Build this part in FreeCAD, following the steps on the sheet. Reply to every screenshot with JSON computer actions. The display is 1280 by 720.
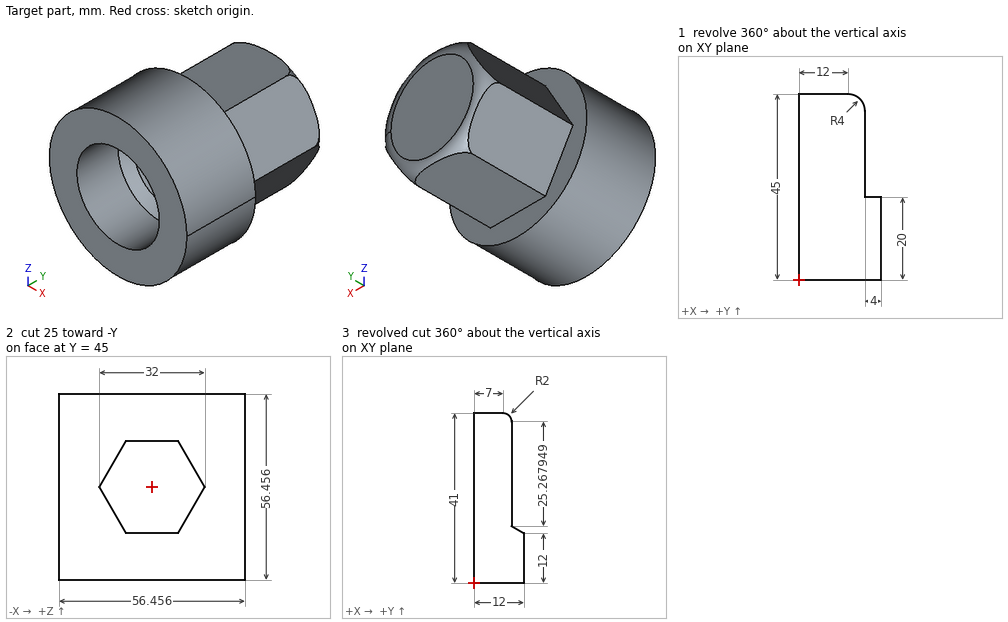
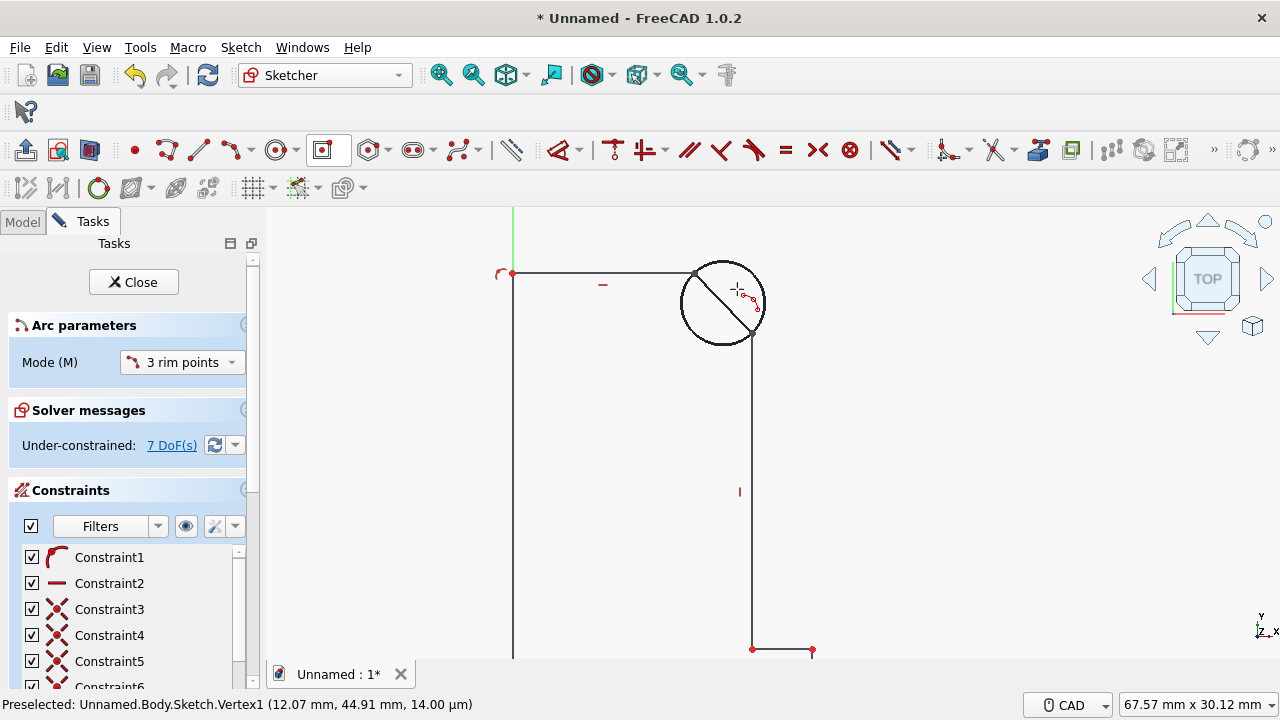
{"action": "left_click", "coordinate": [736, 289]}
{"action": "key", "text": "Escape"}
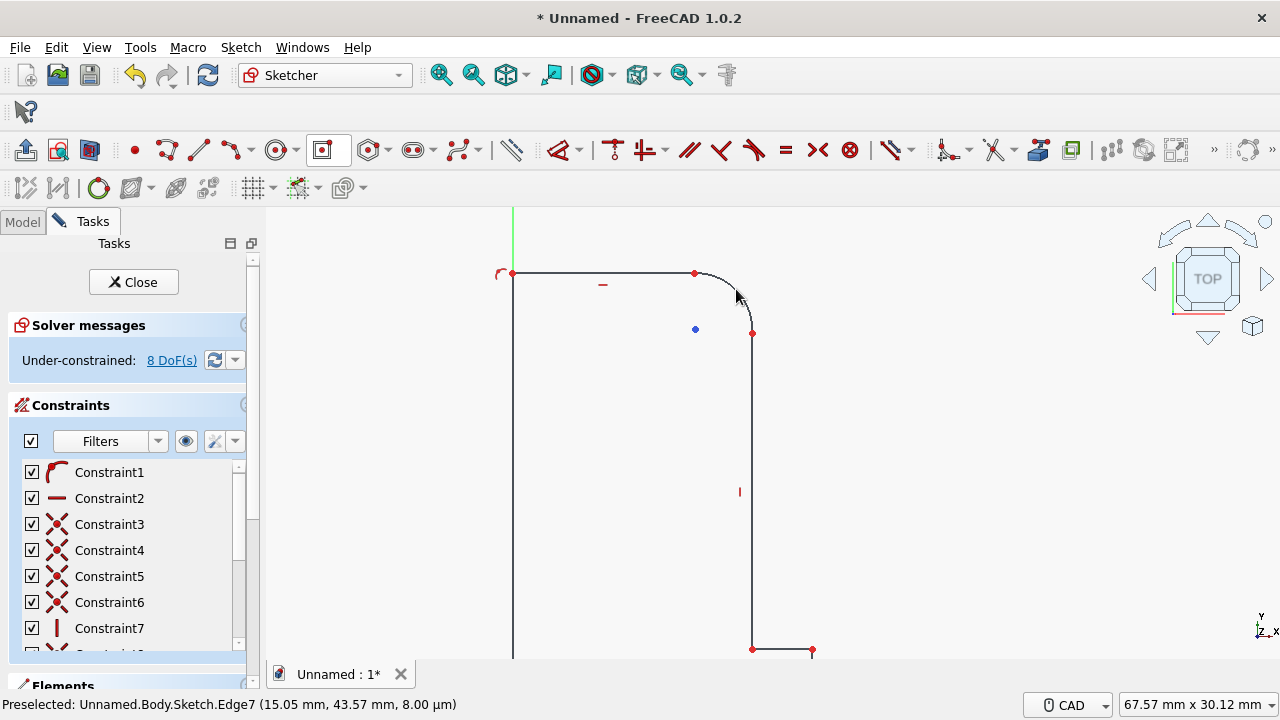
{"action": "left_click", "coordinate": [640, 273]}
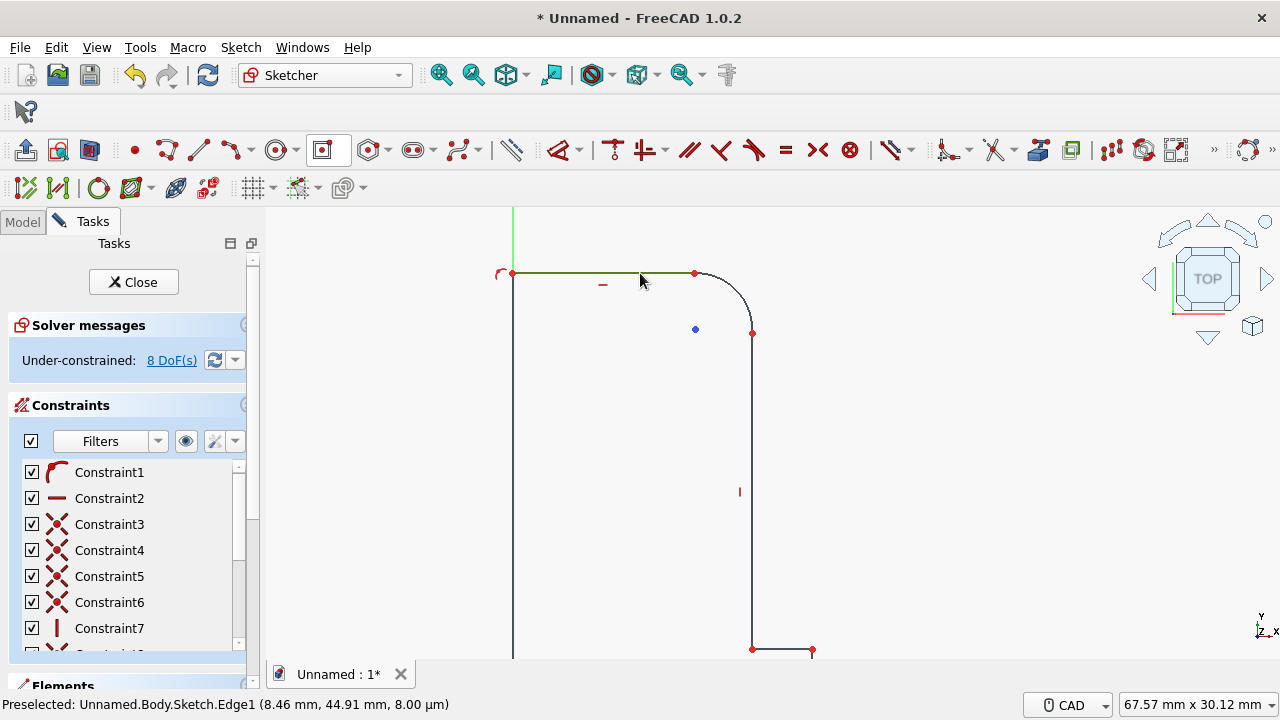
{"action": "left_click", "coordinate": [747, 306]}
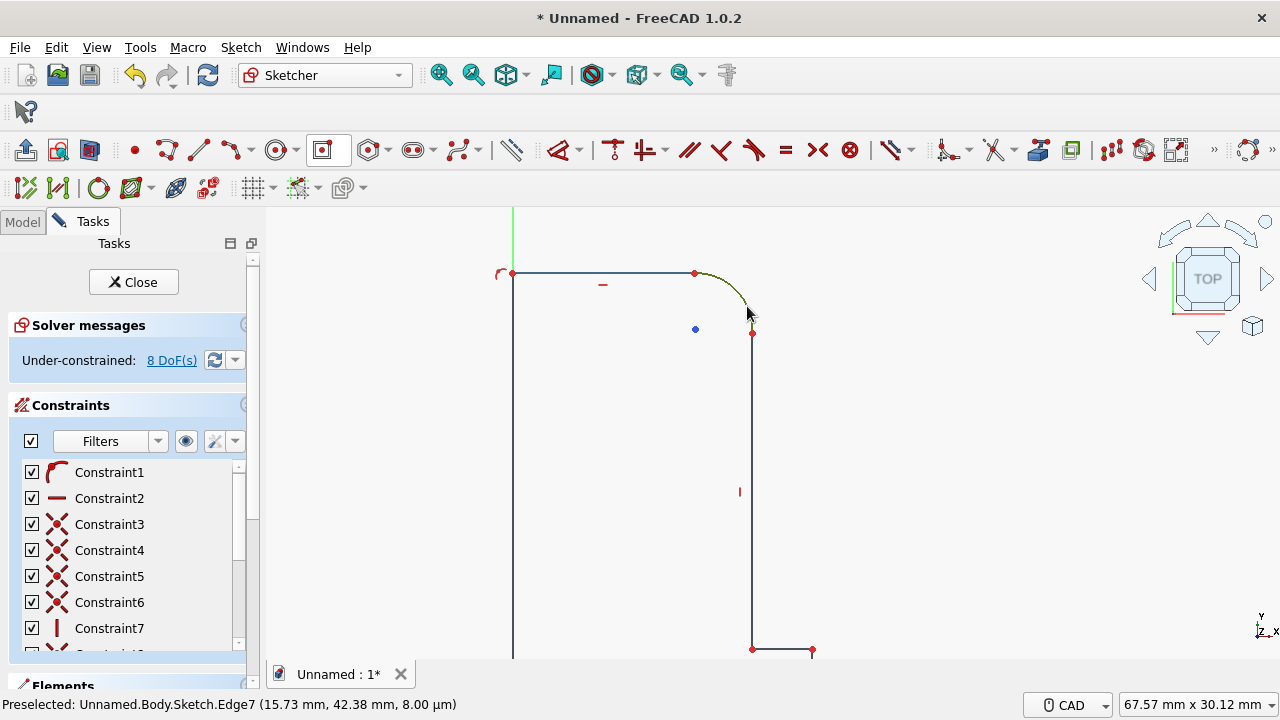
{"action": "key", "text": "t"}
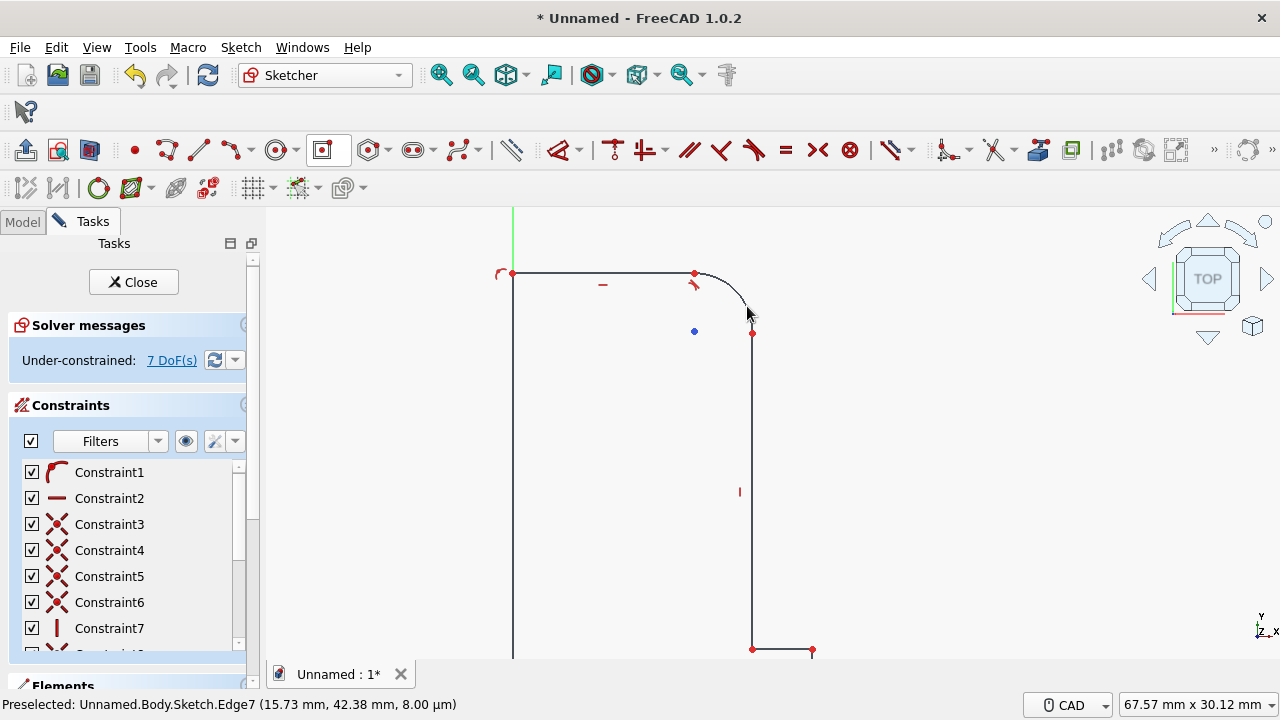
{"action": "left_click", "coordinate": [752, 555]}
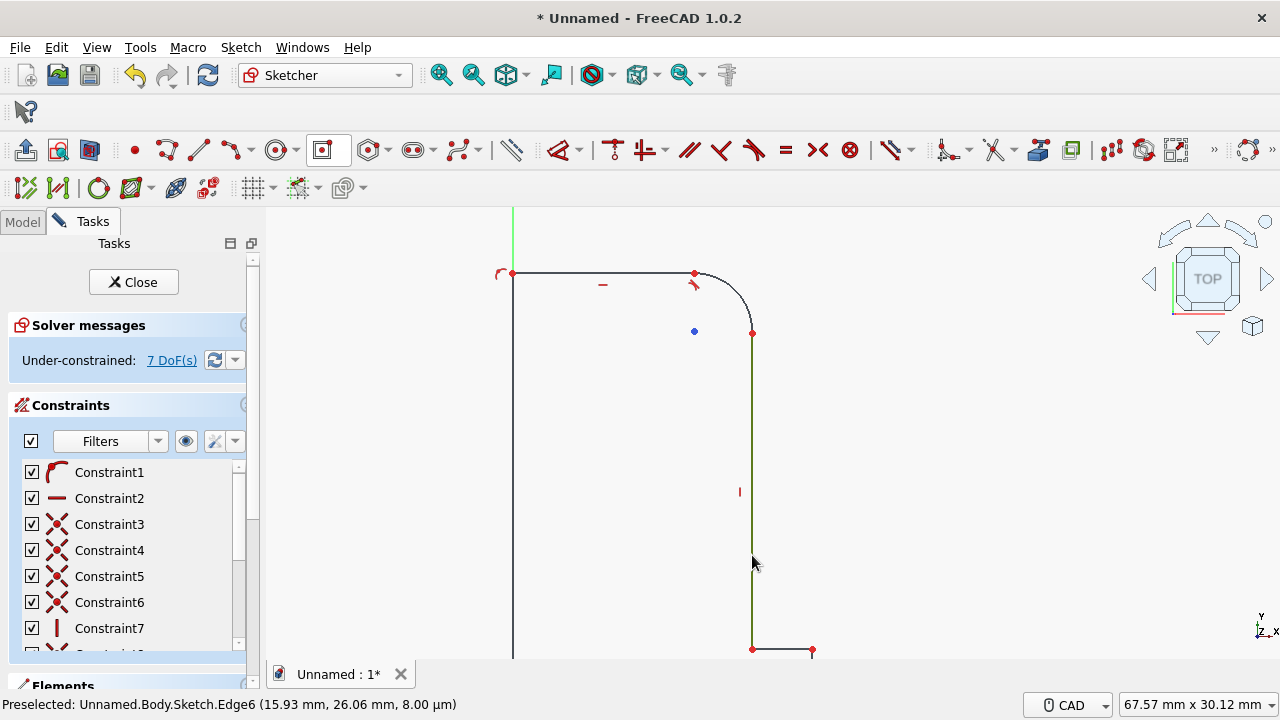
{"action": "left_click", "coordinate": [746, 306]}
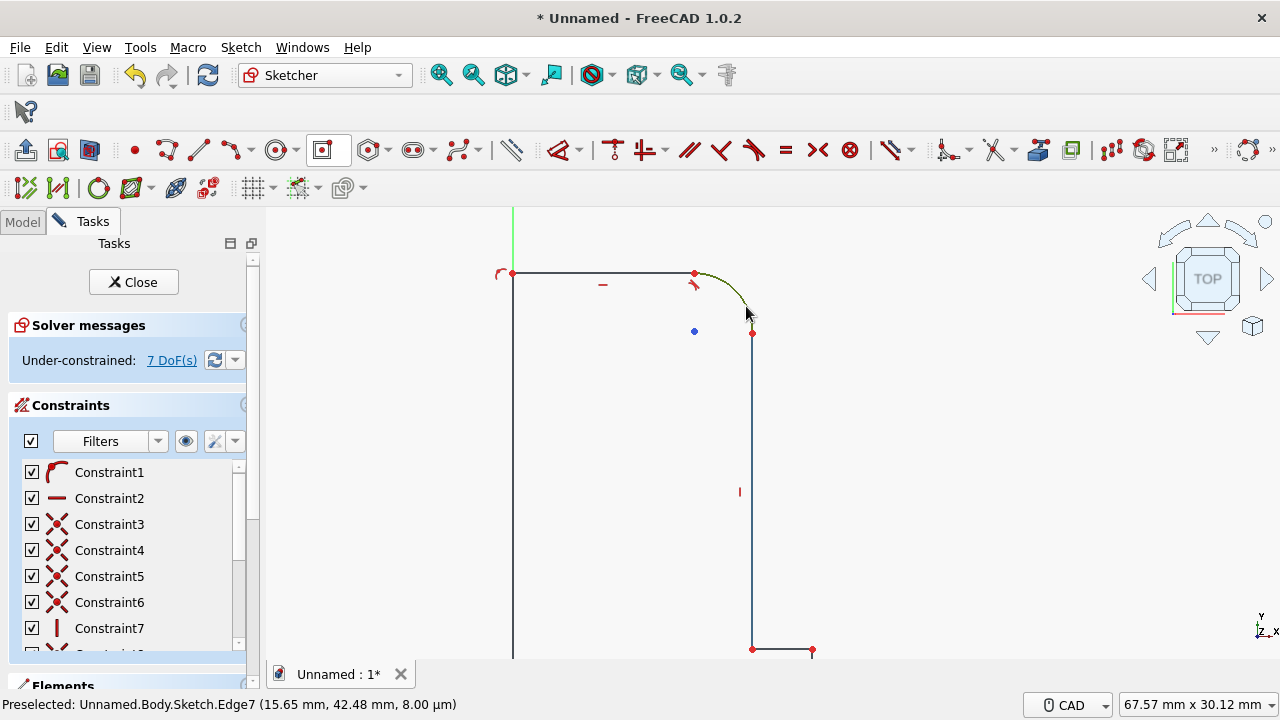
{"action": "key", "text": "t"}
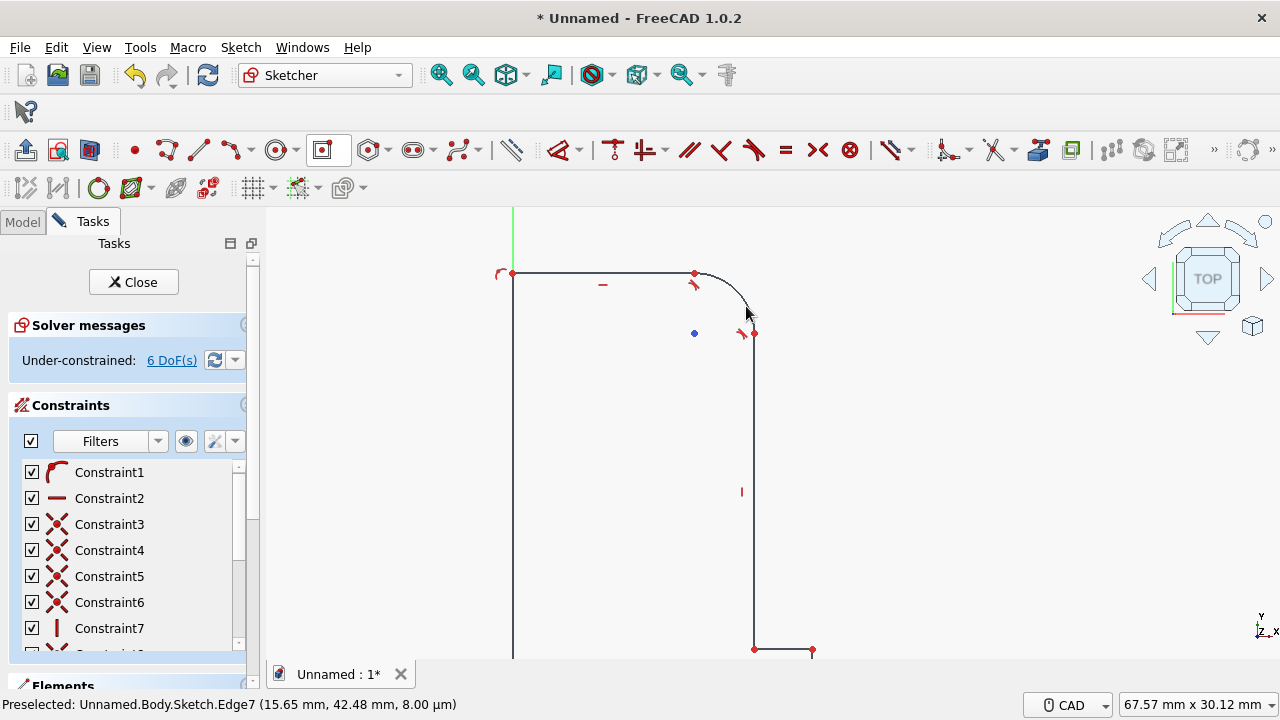
{"action": "scroll", "coordinate": [738, 289], "scroll_direction": "down", "scroll_amount": 4}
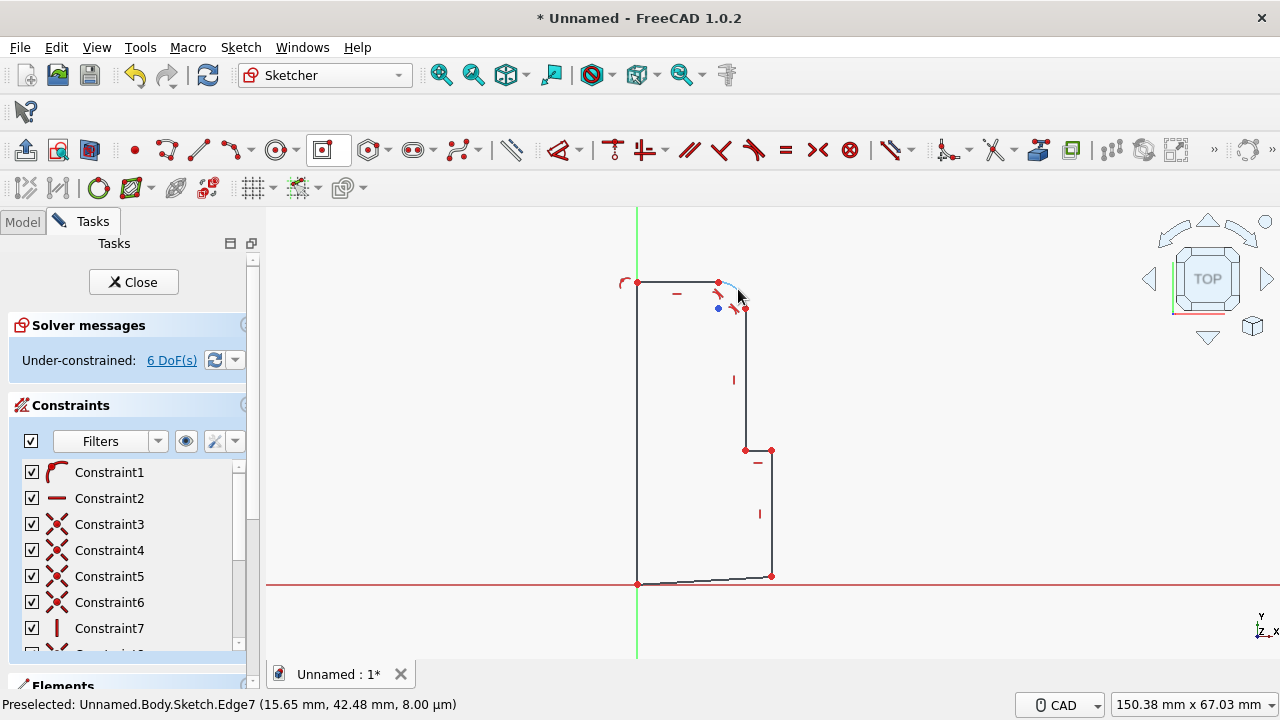
{"action": "scroll", "coordinate": [731, 579], "scroll_direction": "up", "scroll_amount": 5}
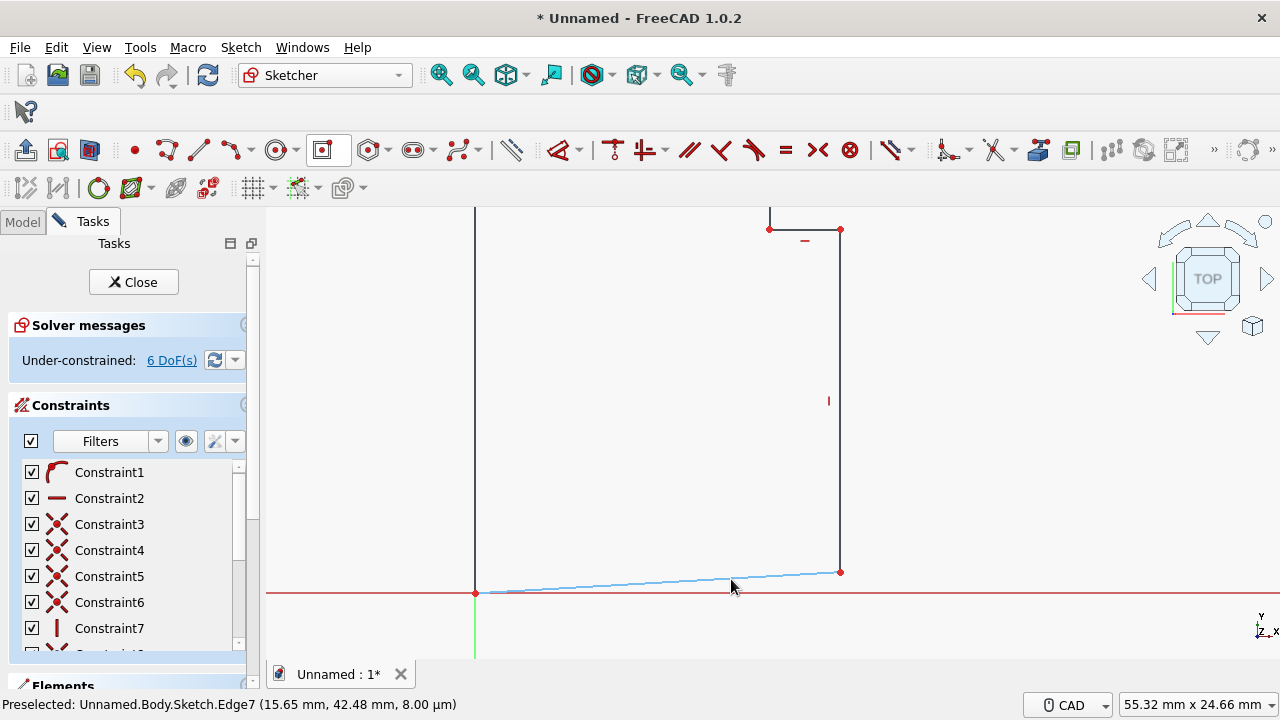
{"action": "left_click", "coordinate": [731, 579]}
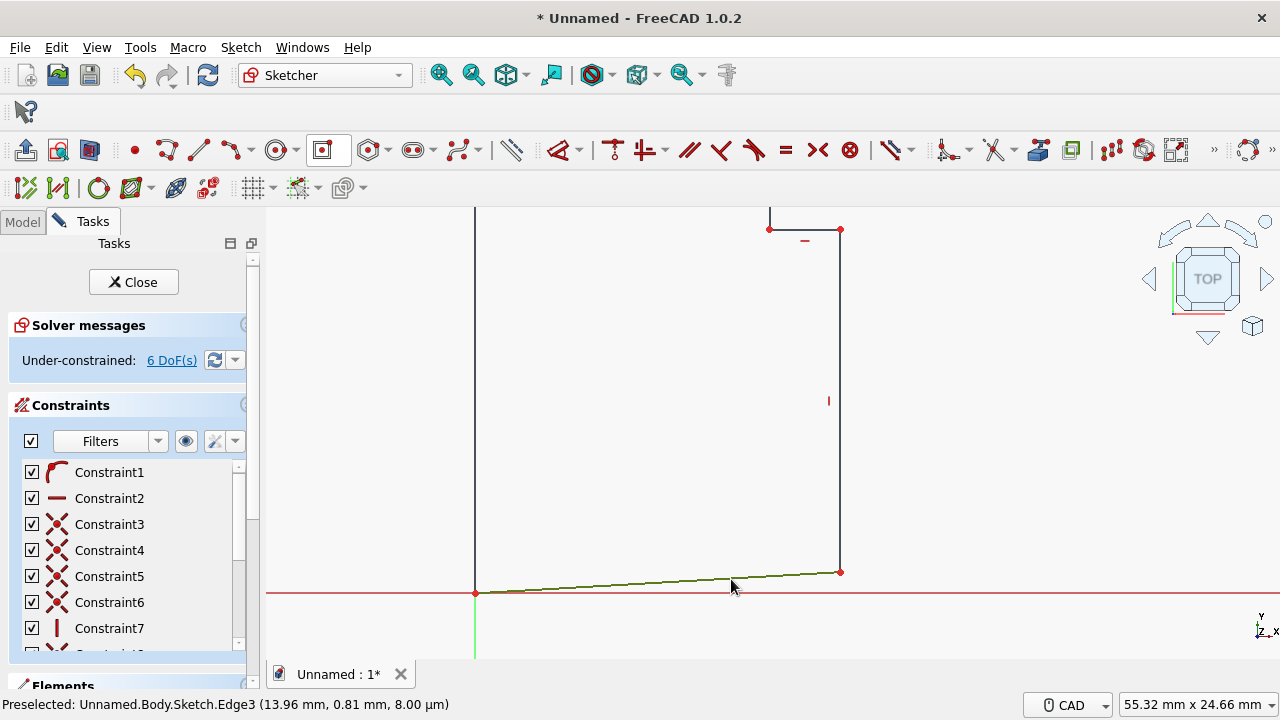
{"action": "key", "text": "h"}